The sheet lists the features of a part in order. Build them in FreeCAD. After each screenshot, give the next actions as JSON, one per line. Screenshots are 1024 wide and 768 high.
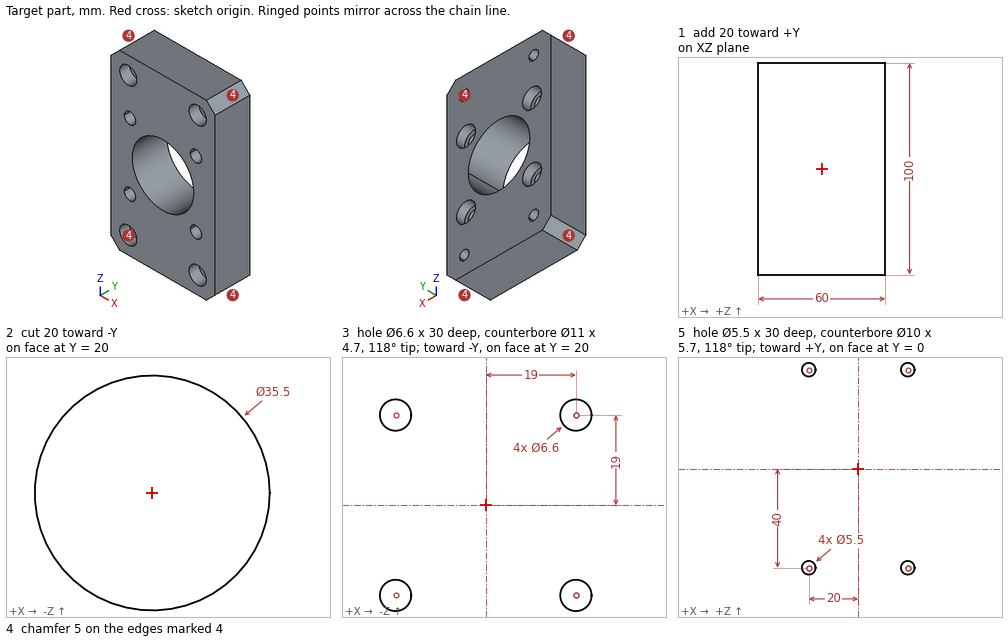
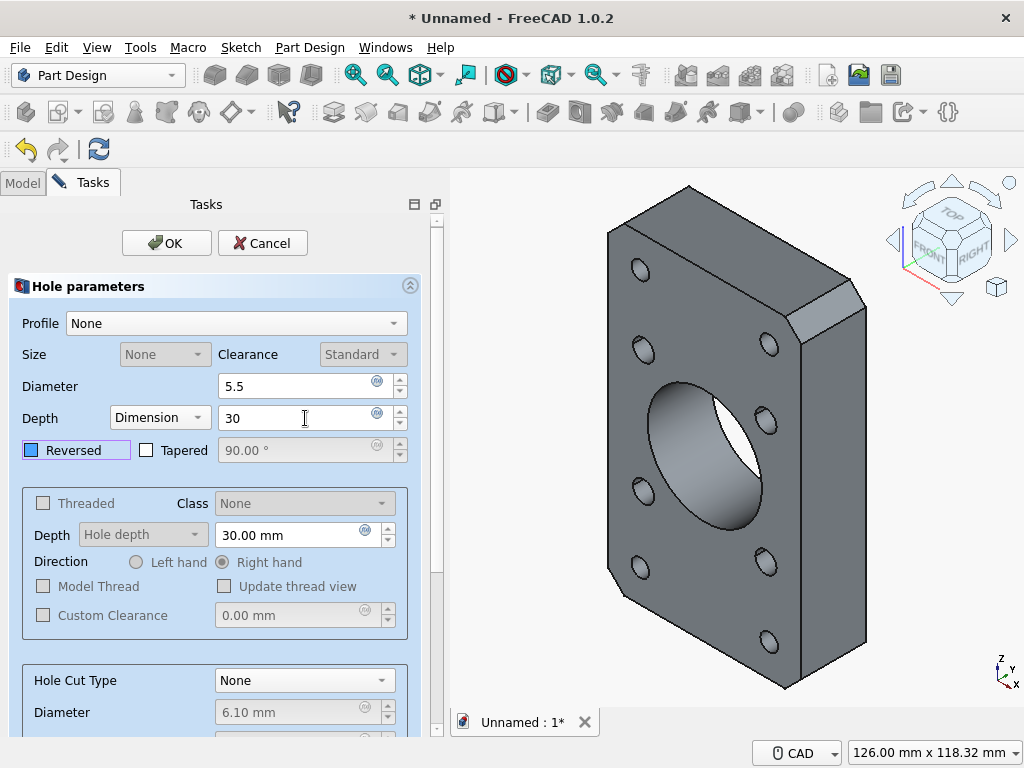
{"action": "left_click", "coordinate": [306, 680]}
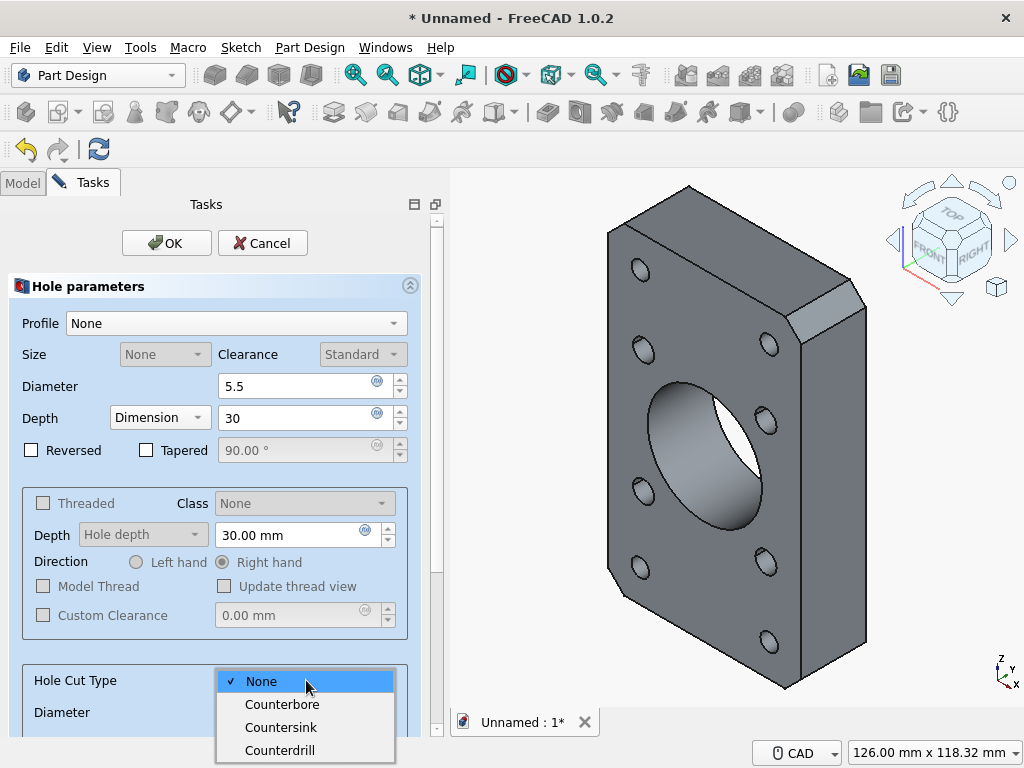
{"action": "left_click", "coordinate": [304, 704]}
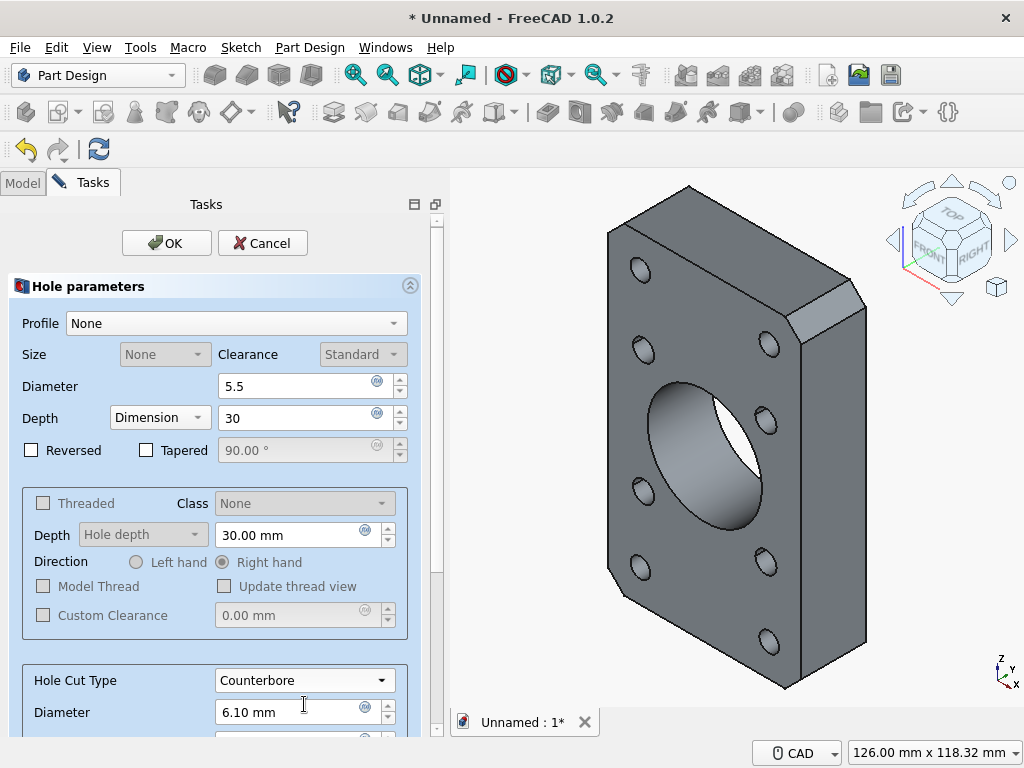
{"action": "triple_click", "coordinate": [298, 712]}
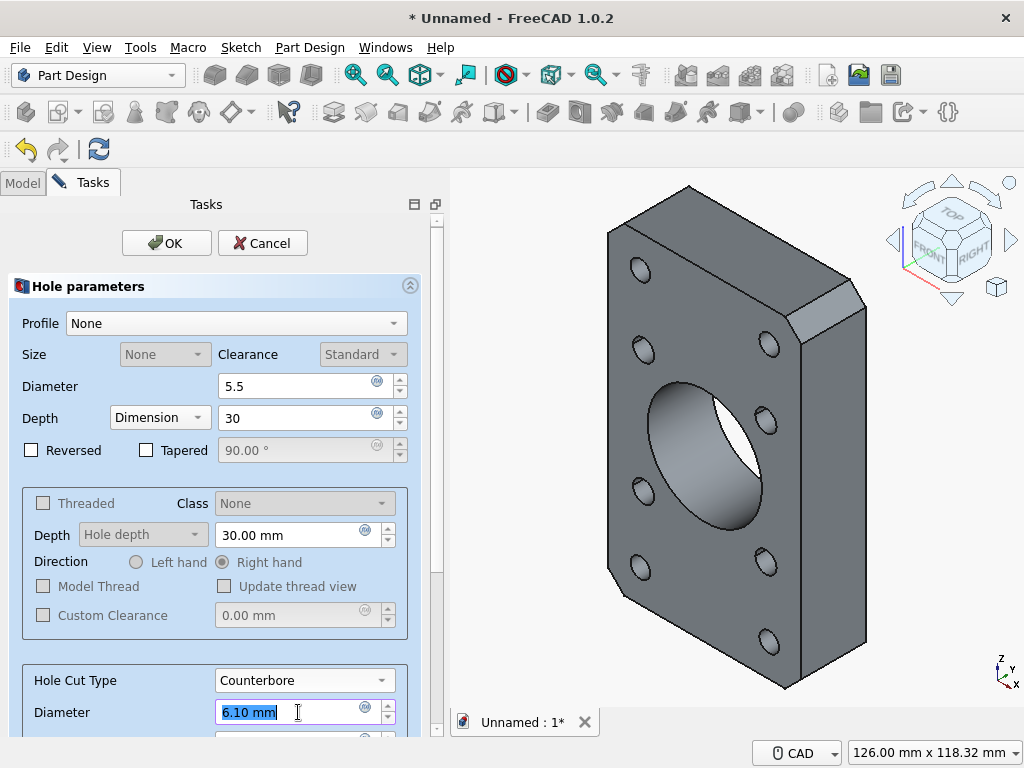
{"action": "type", "text": "10"}
{"action": "key", "text": "Tab"}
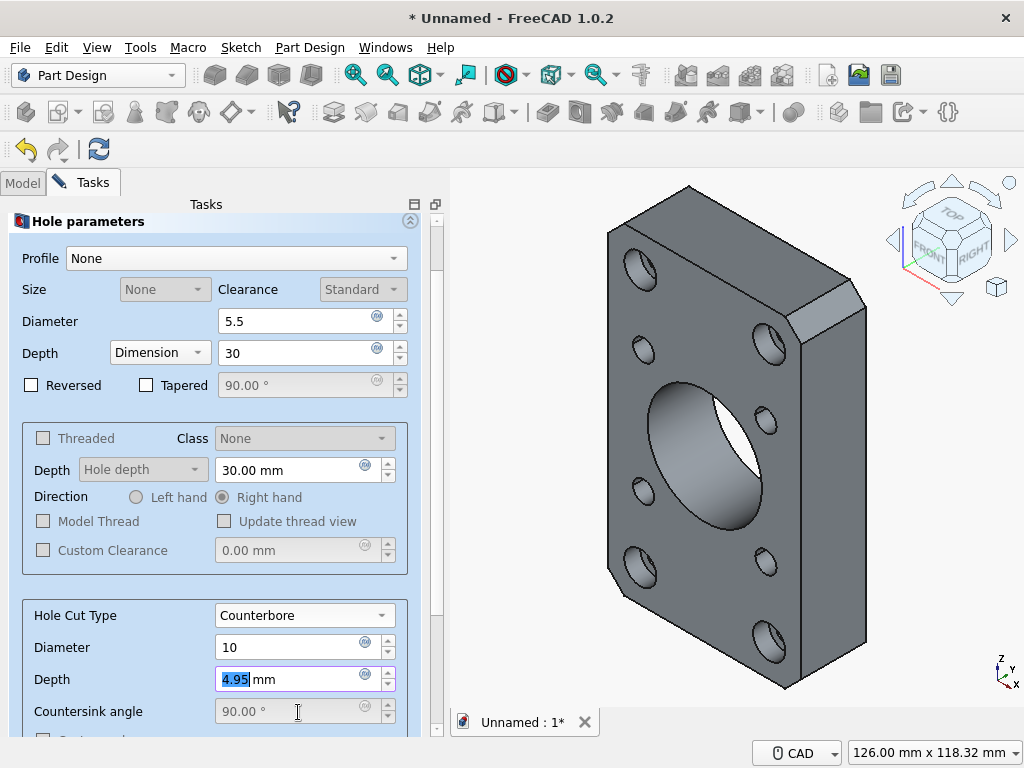
{"action": "type", "text": "5.7"}
{"action": "key", "text": "Tab"}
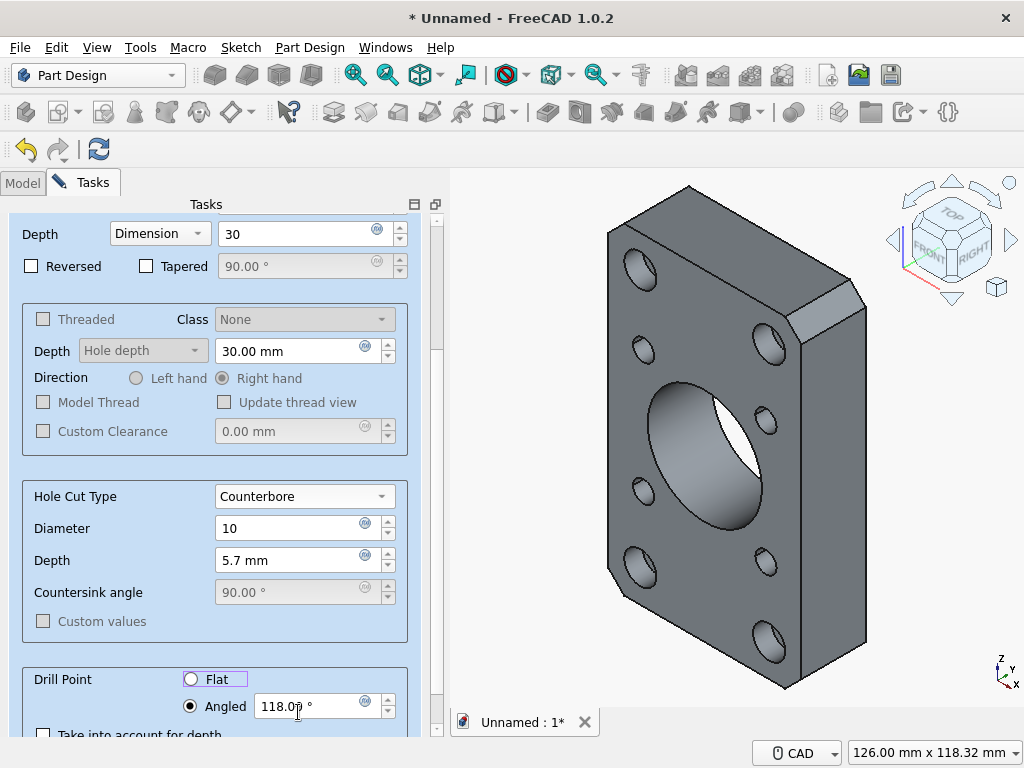
{"action": "scroll", "coordinate": [437, 475], "scroll_direction": "up", "scroll_amount": 4}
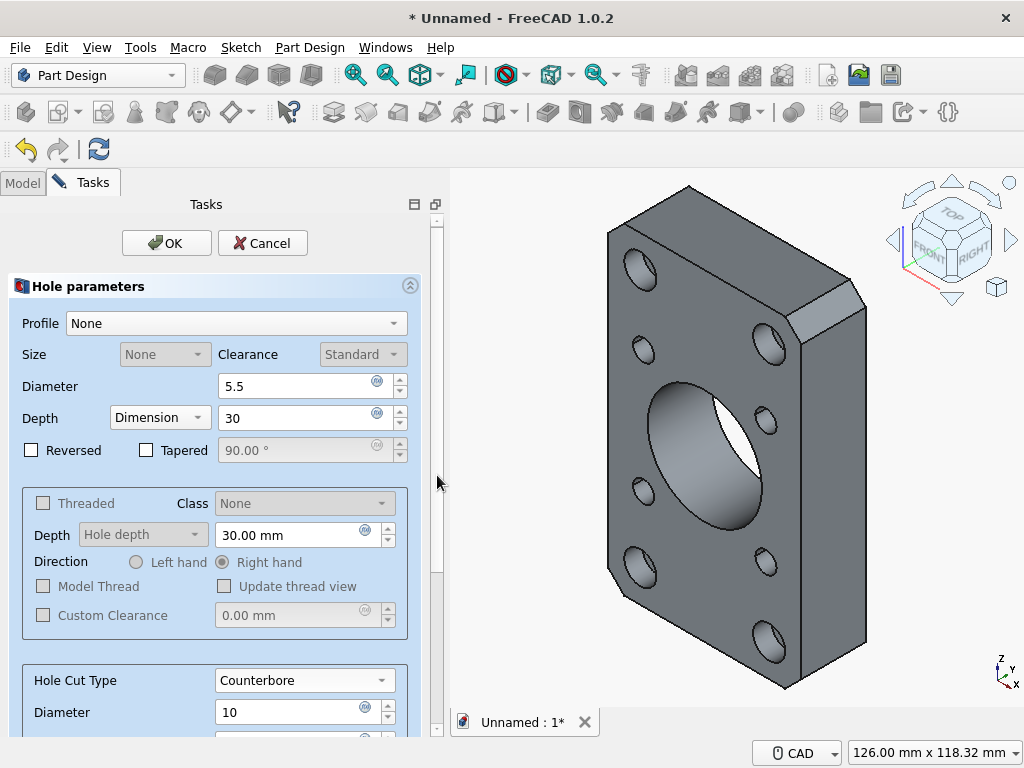
{"action": "left_click", "coordinate": [167, 243]}